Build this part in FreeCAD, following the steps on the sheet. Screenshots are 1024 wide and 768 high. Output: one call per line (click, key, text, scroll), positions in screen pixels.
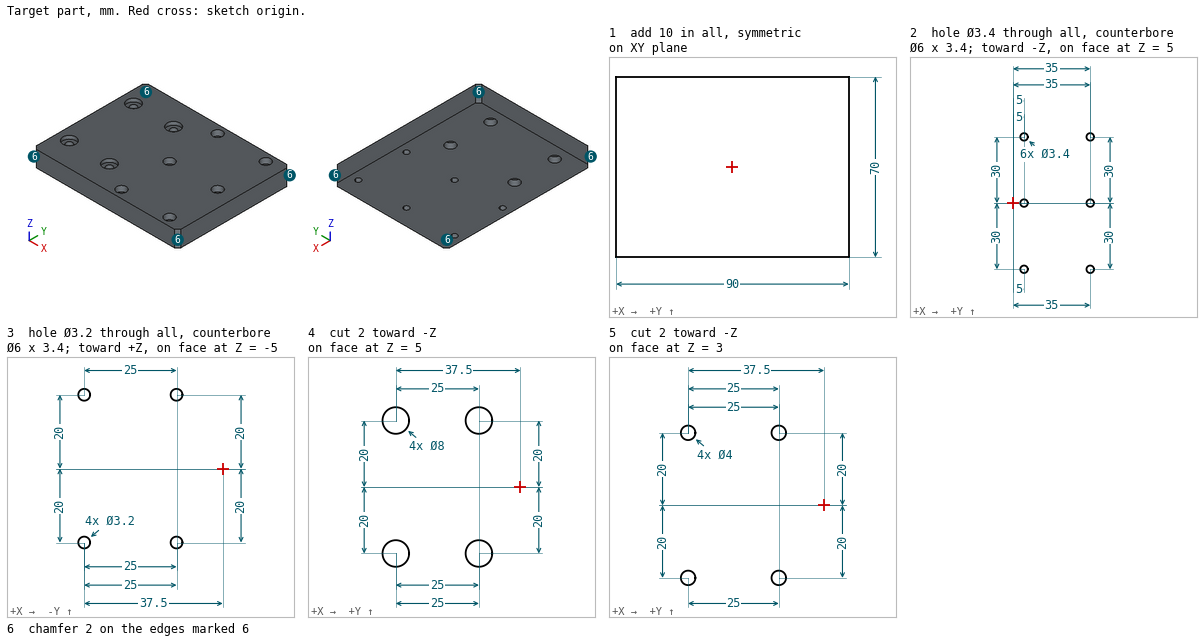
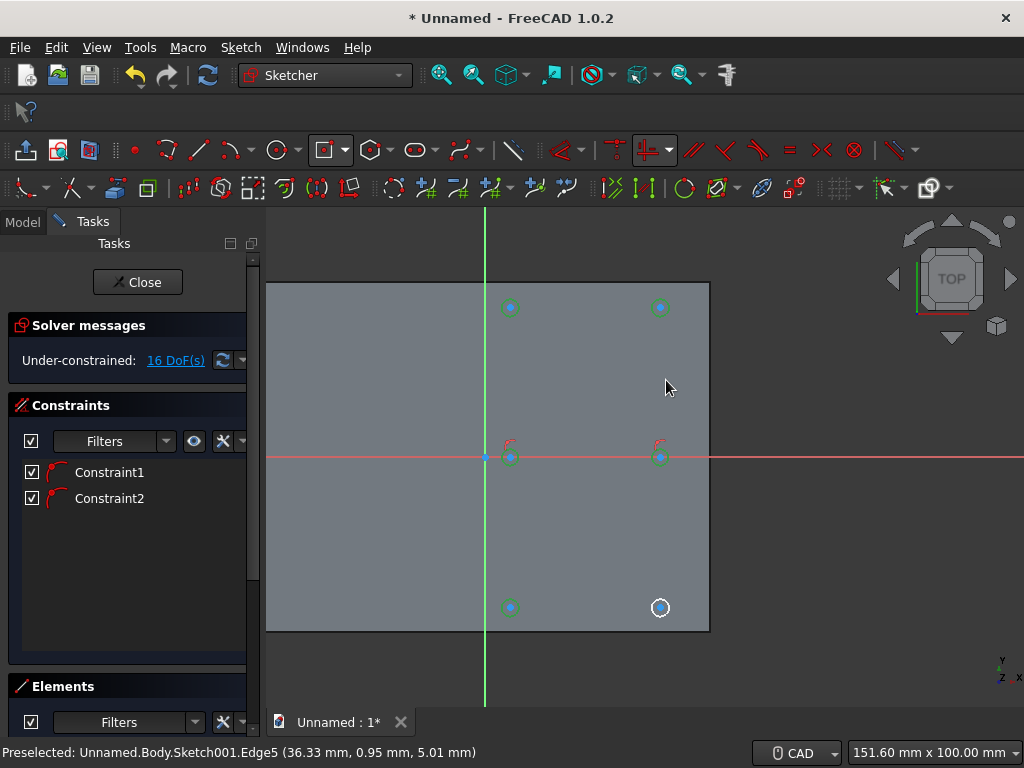
scroll(666, 602, up, 3)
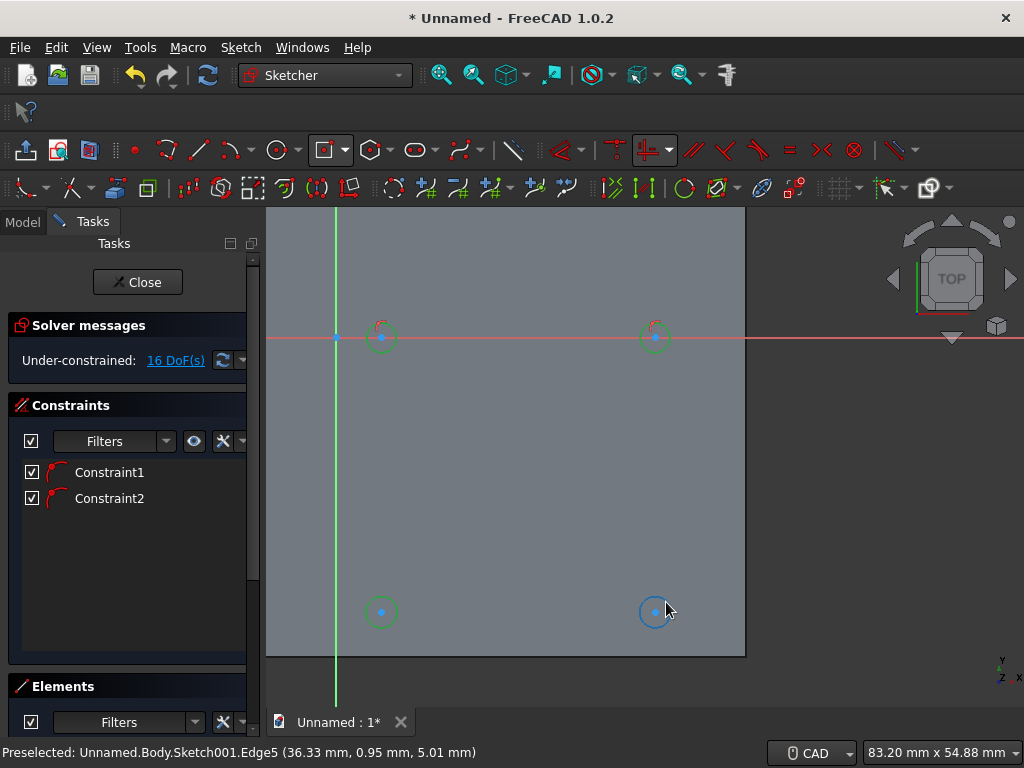
click(666, 601)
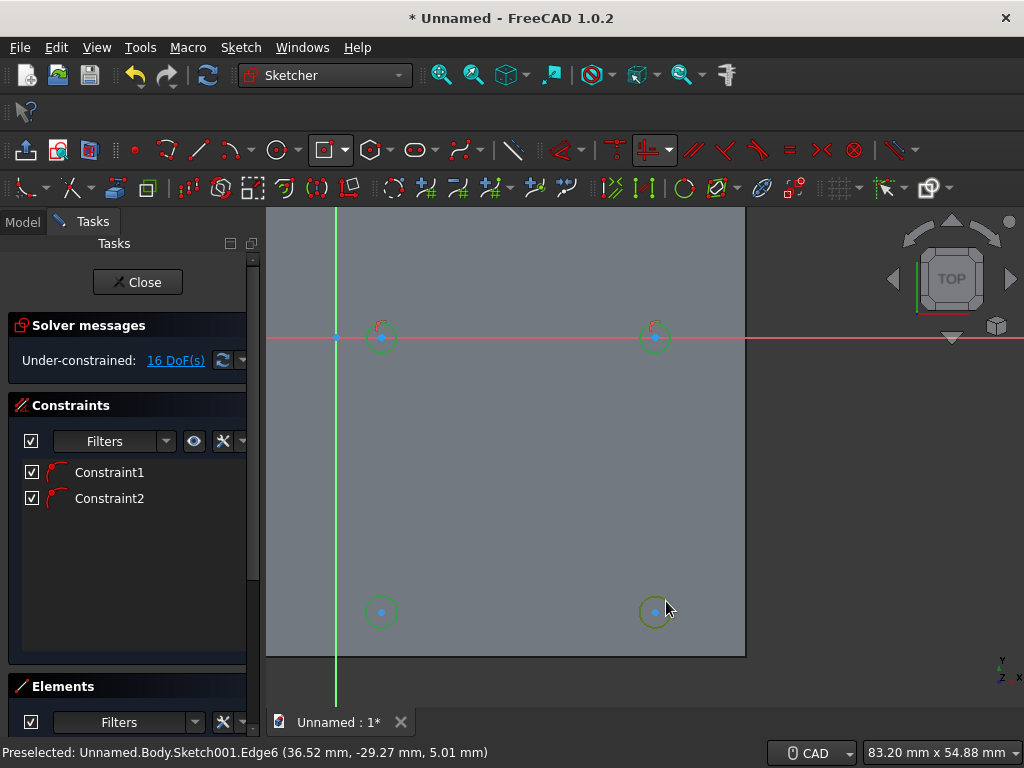
click(790, 150)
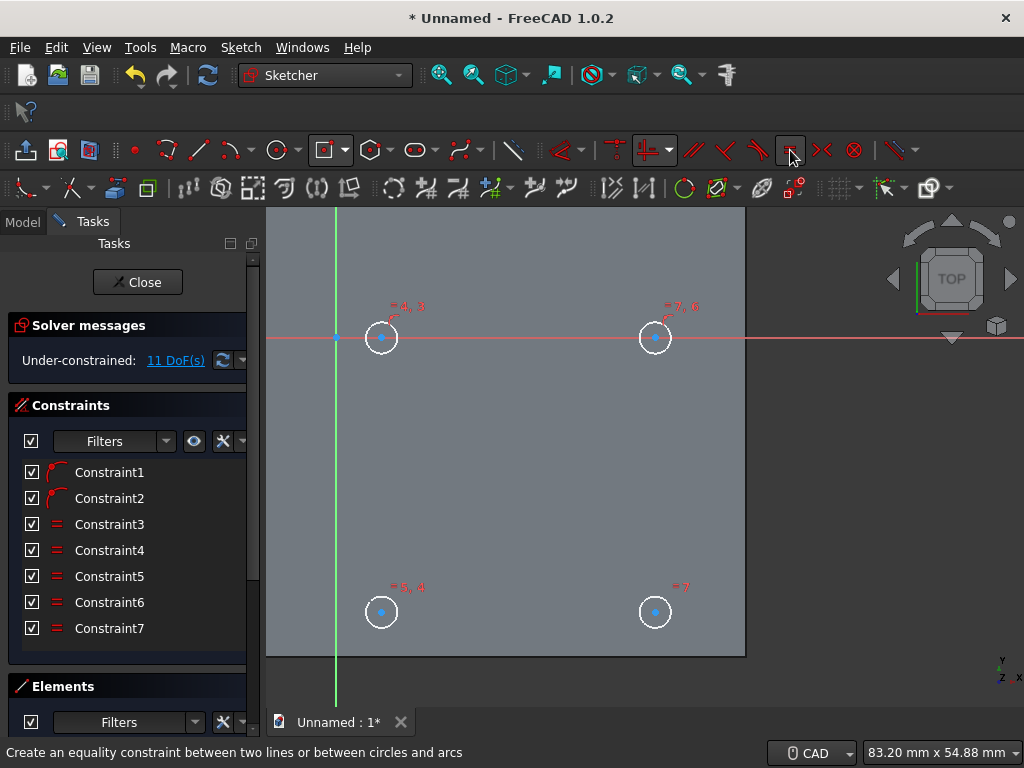
click(560, 150)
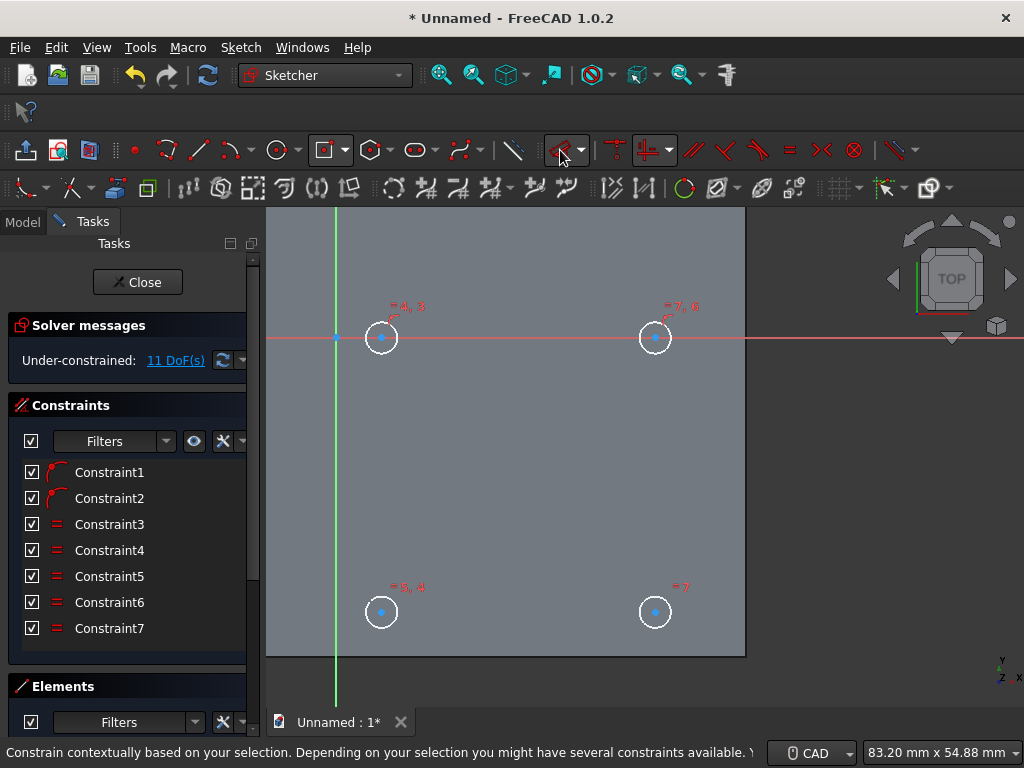
scroll(665, 602, down, 3)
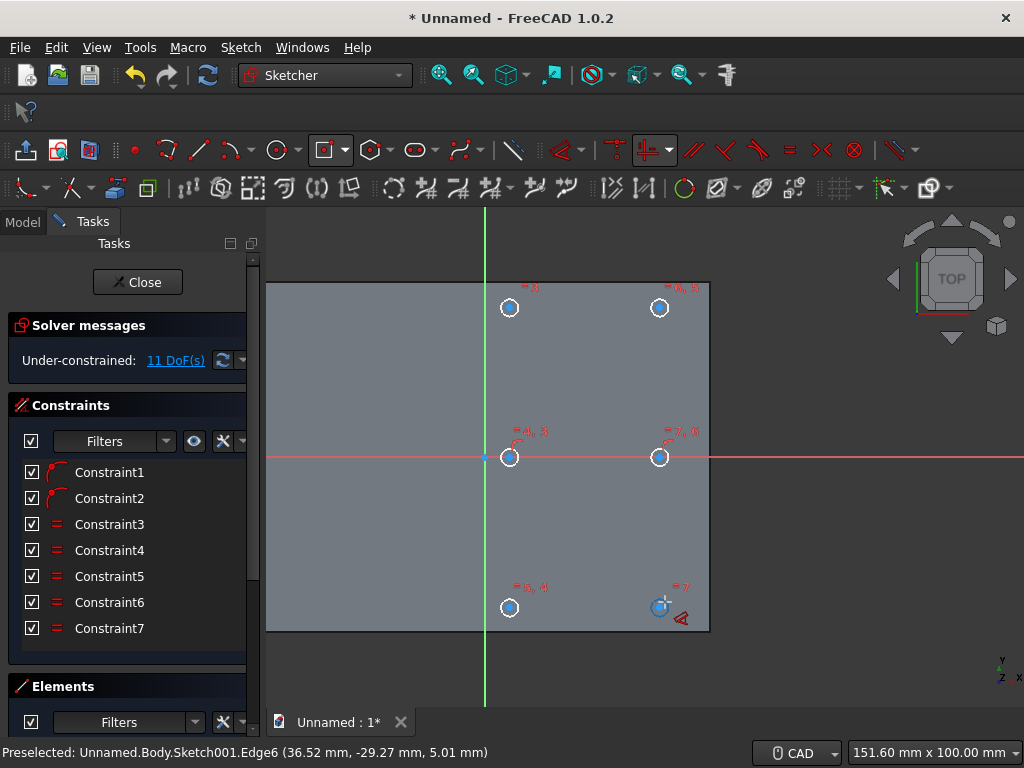
scroll(516, 302, up, 5)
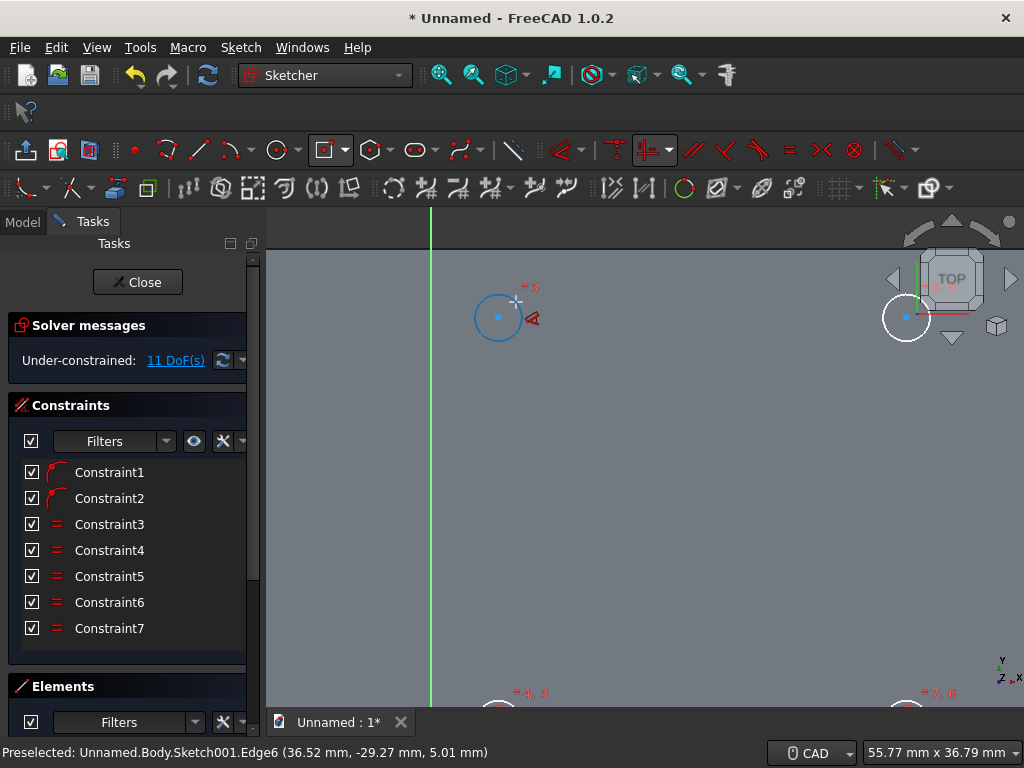
click(515, 301)
click(537, 278)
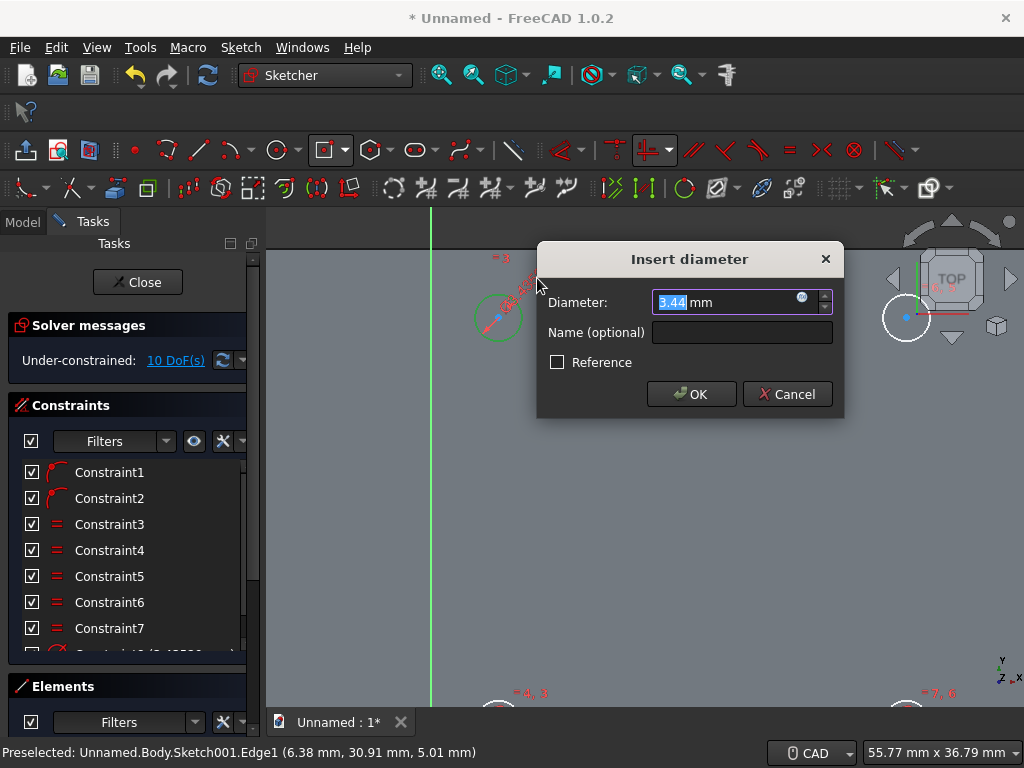
text(3.4)
key(Return)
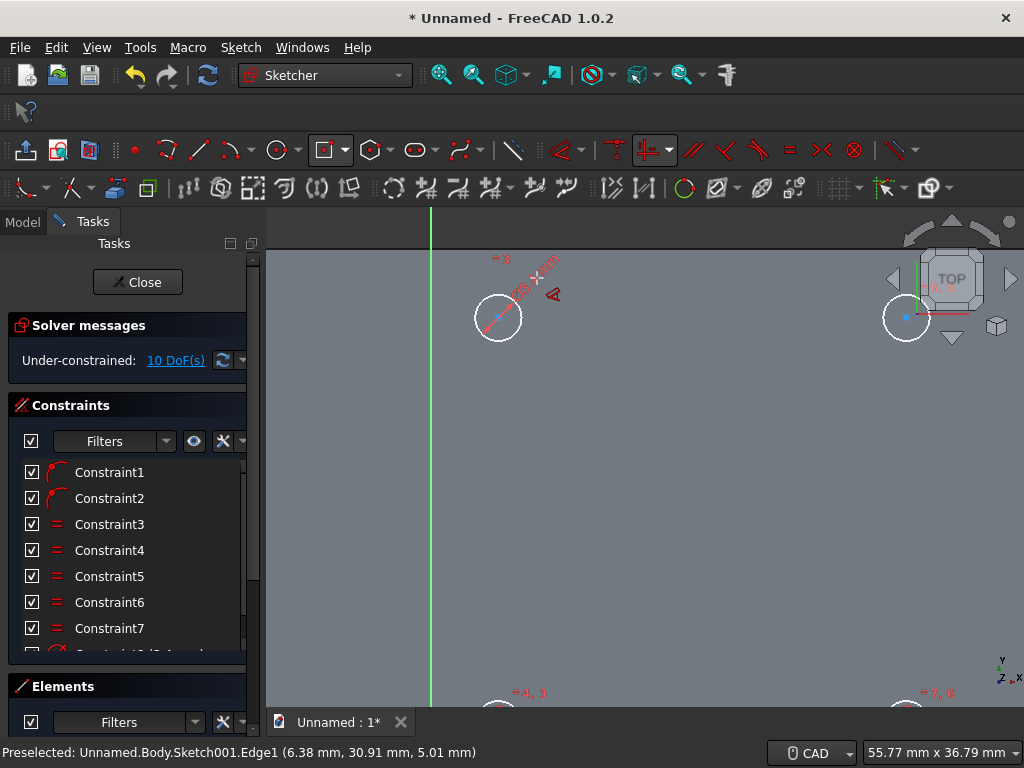
click(498, 318)
click(464, 284)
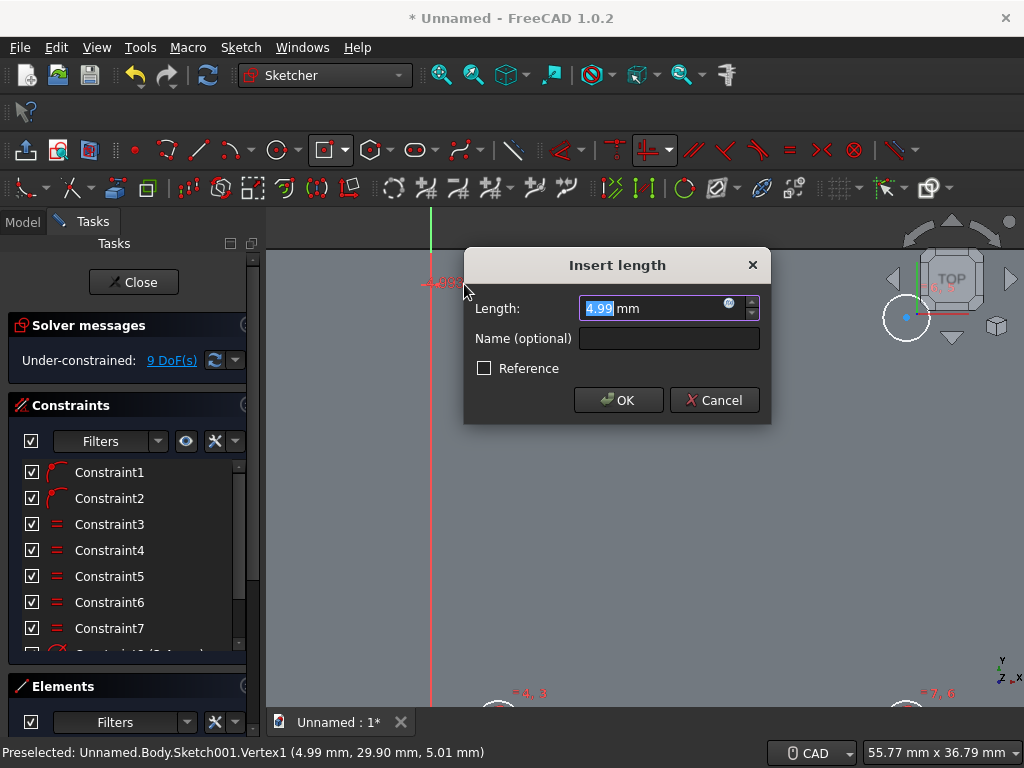
text(5)
key(Return)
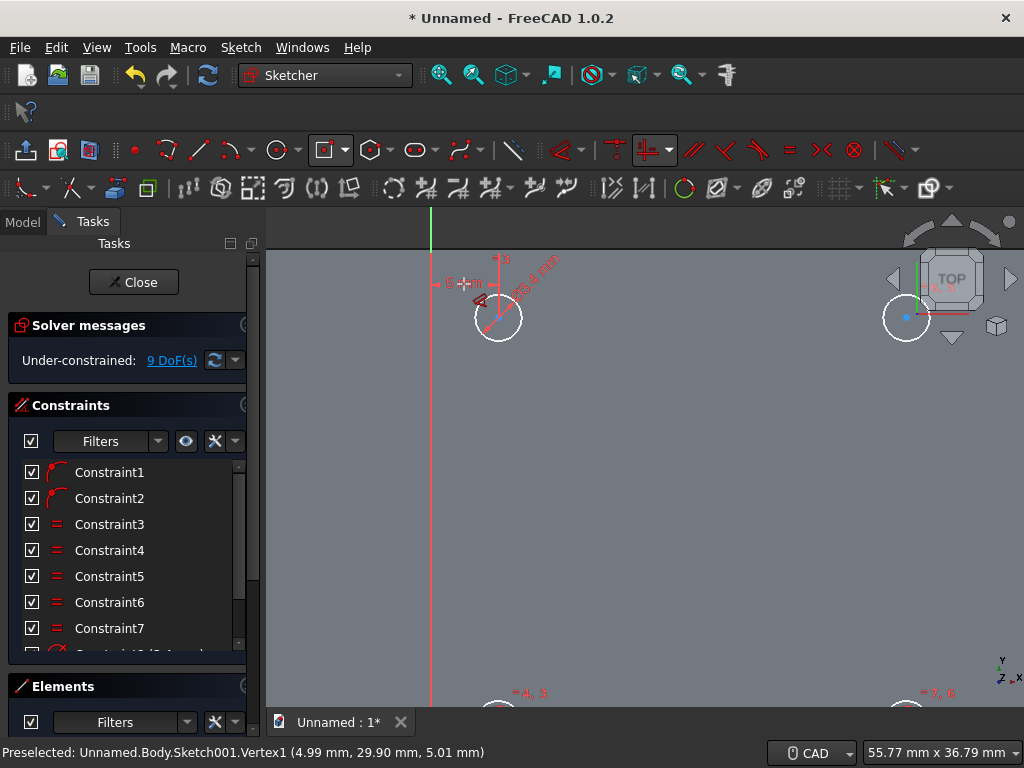
scroll(516, 301, down, 5)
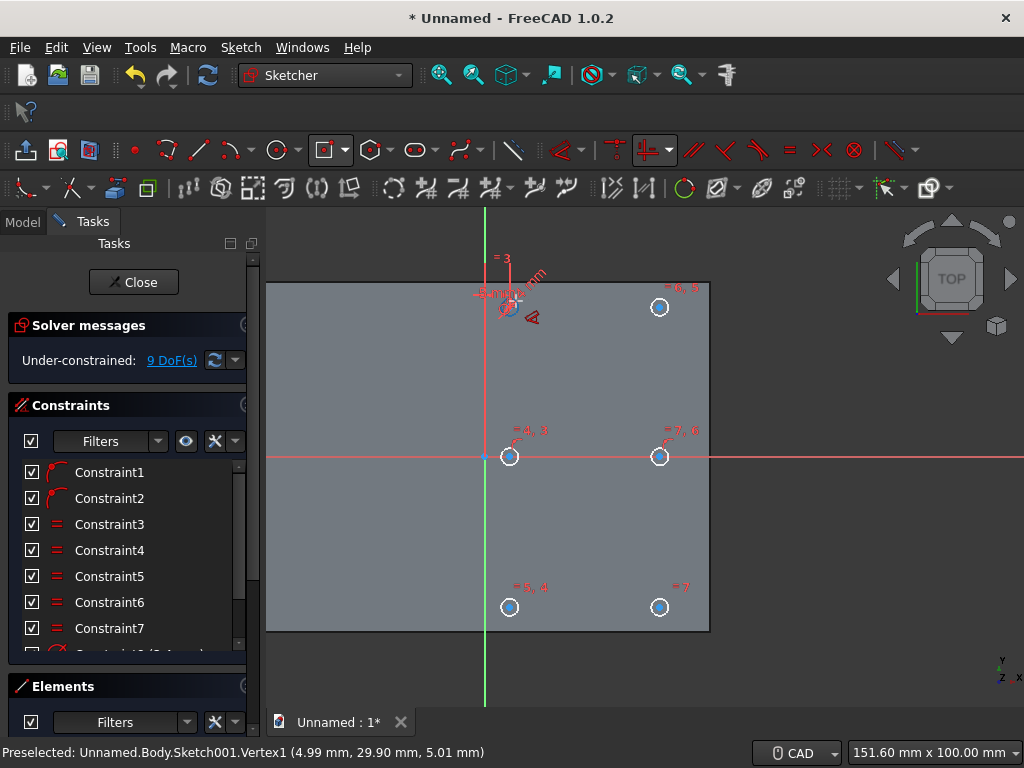
scroll(510, 457, up, 3)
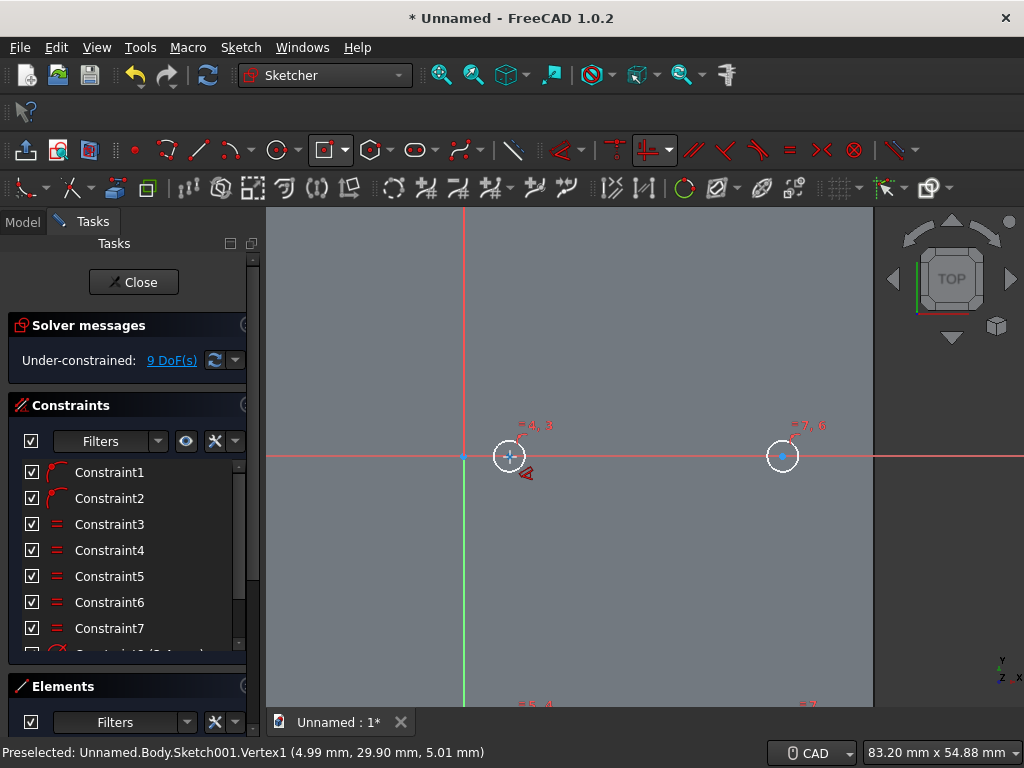
click(509, 456)
click(487, 490)